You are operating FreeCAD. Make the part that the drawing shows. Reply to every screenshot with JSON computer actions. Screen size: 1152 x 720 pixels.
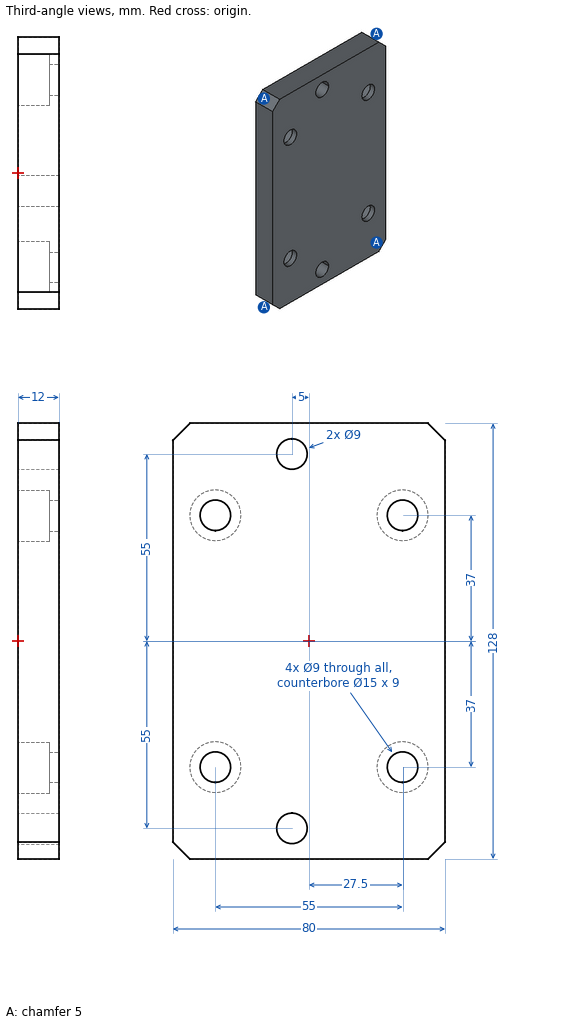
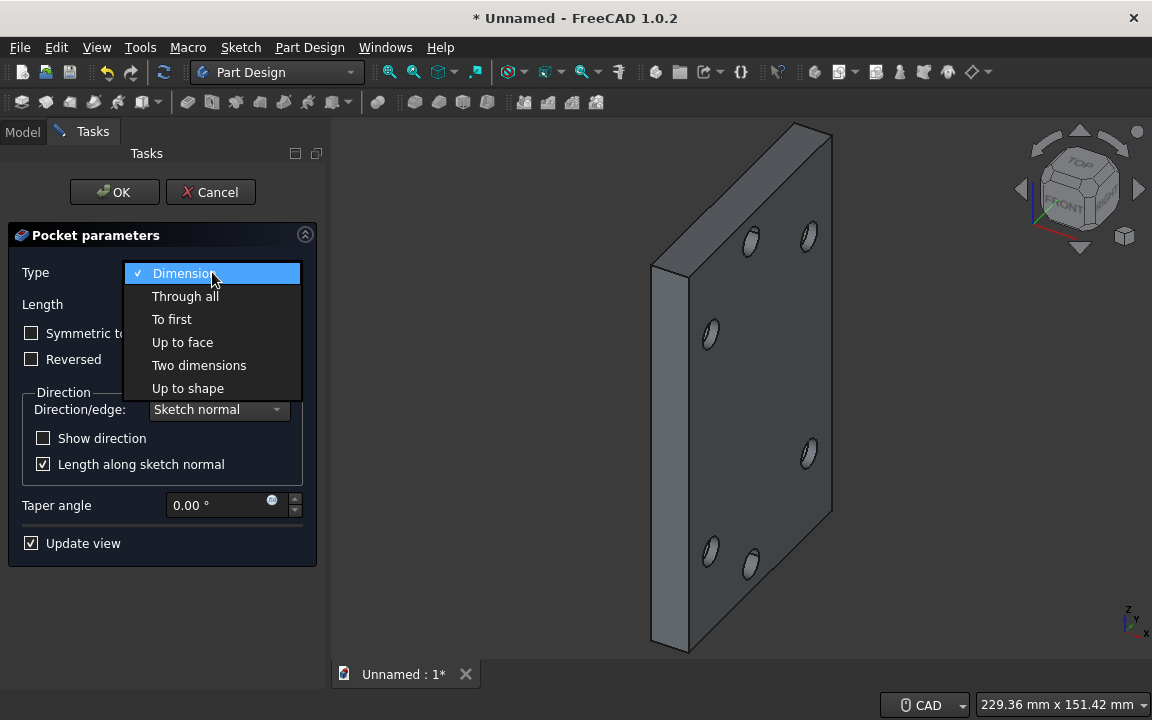
{"action": "left_click", "coordinate": [212, 296]}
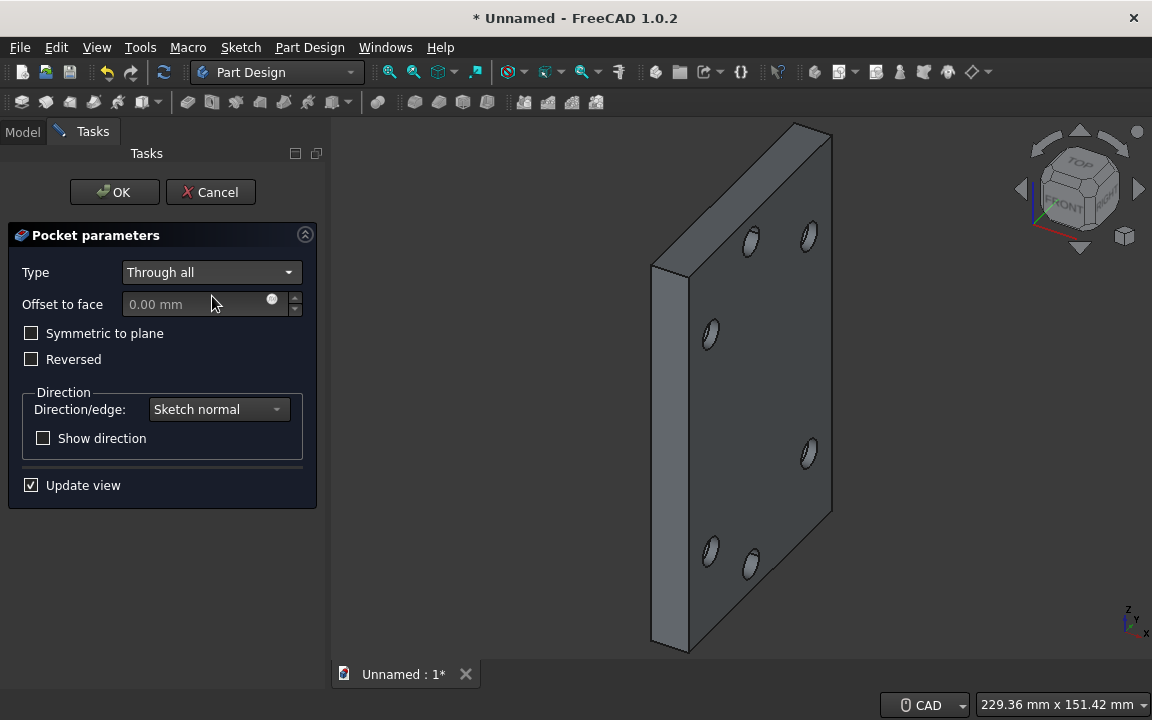
{"action": "left_click", "coordinate": [115, 192]}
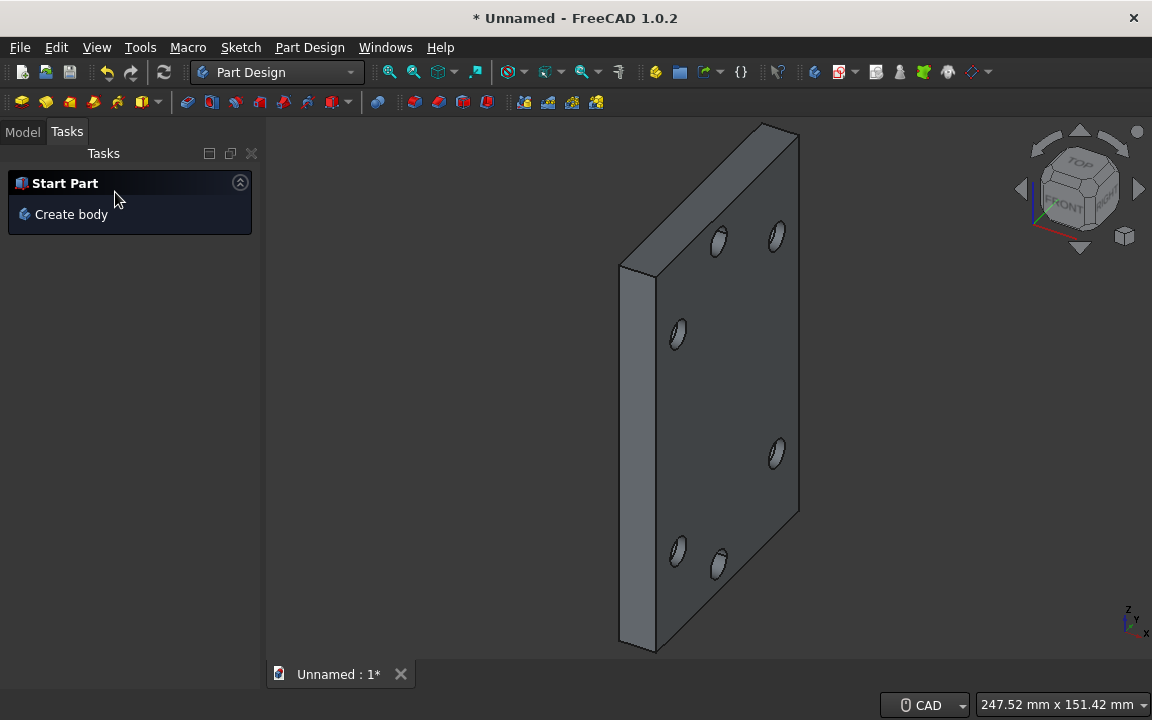
{"action": "left_click", "coordinate": [637, 270]}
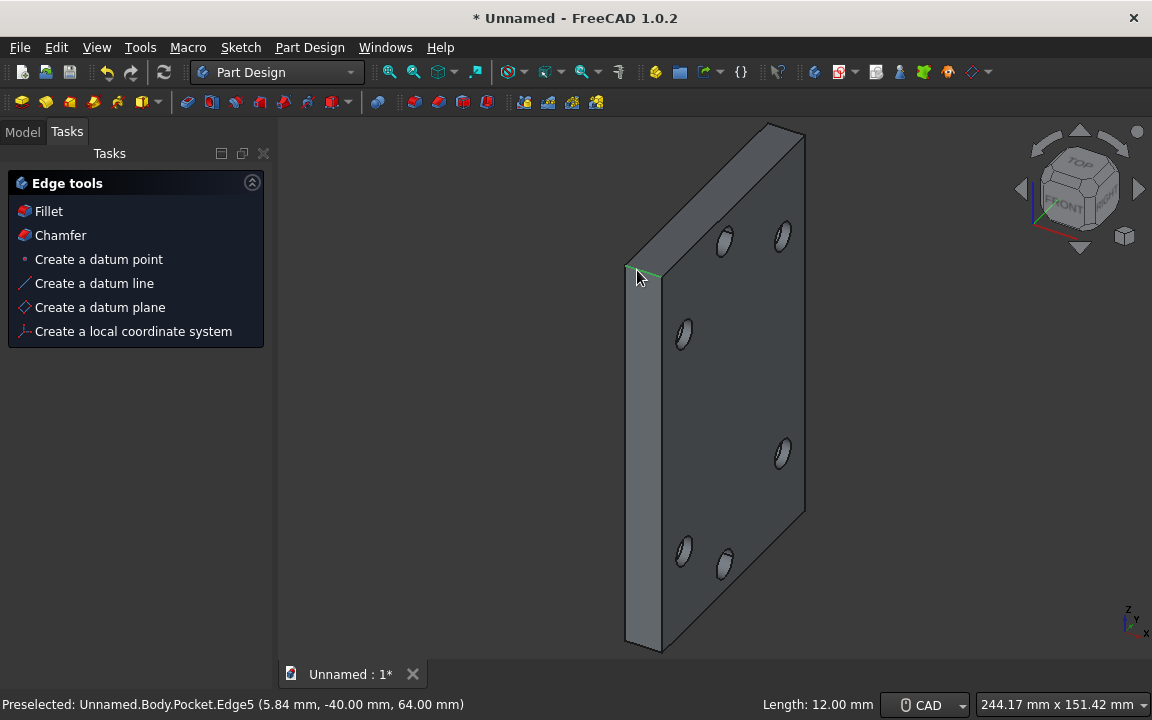
{"action": "key", "text": "0"}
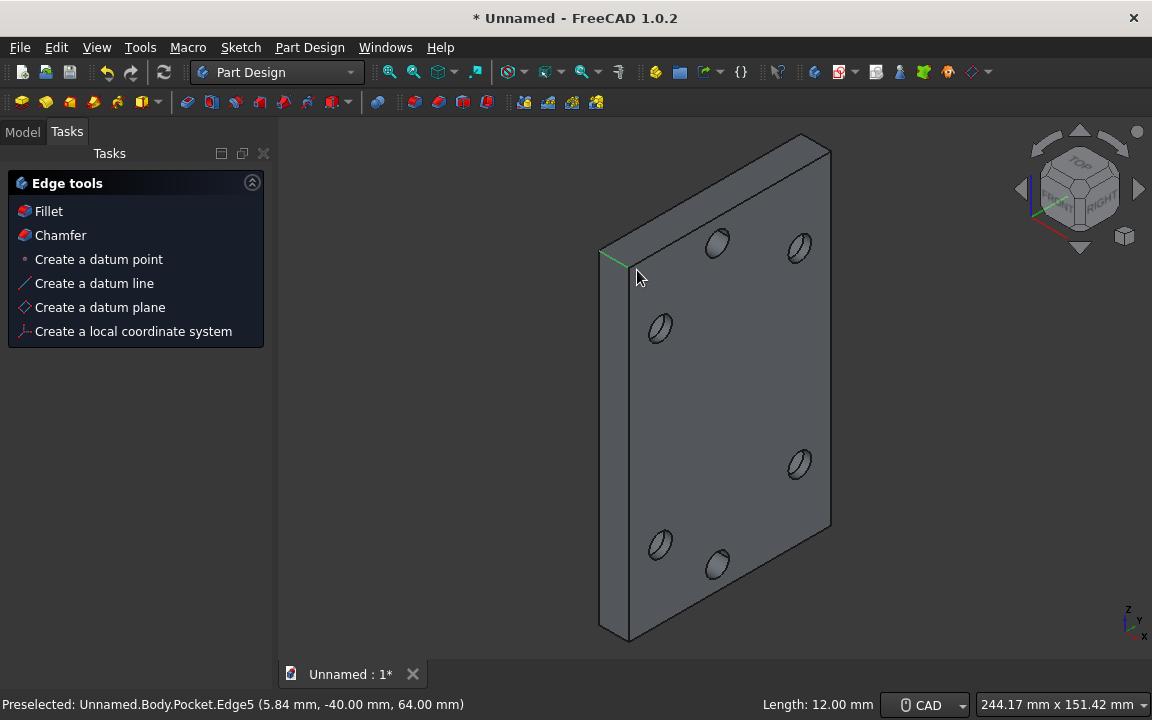
{"action": "key", "text": "2"}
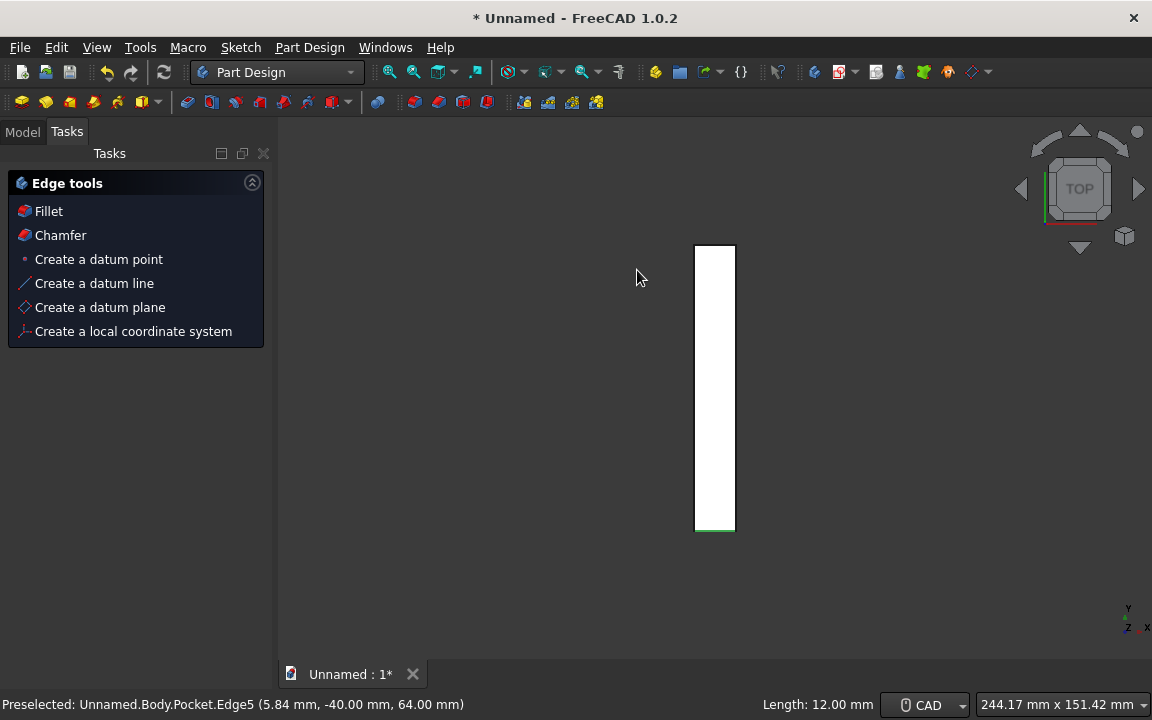
{"action": "left_click", "coordinate": [715, 244], "text": "ctrl"}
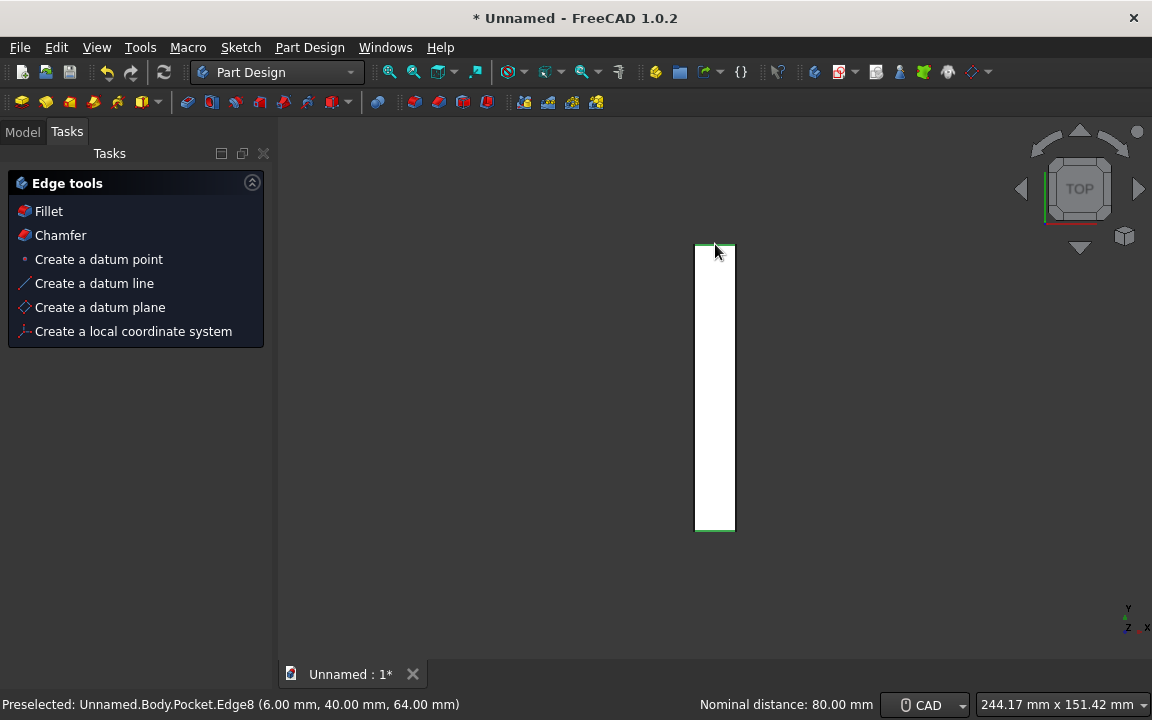
{"action": "key", "text": "1"}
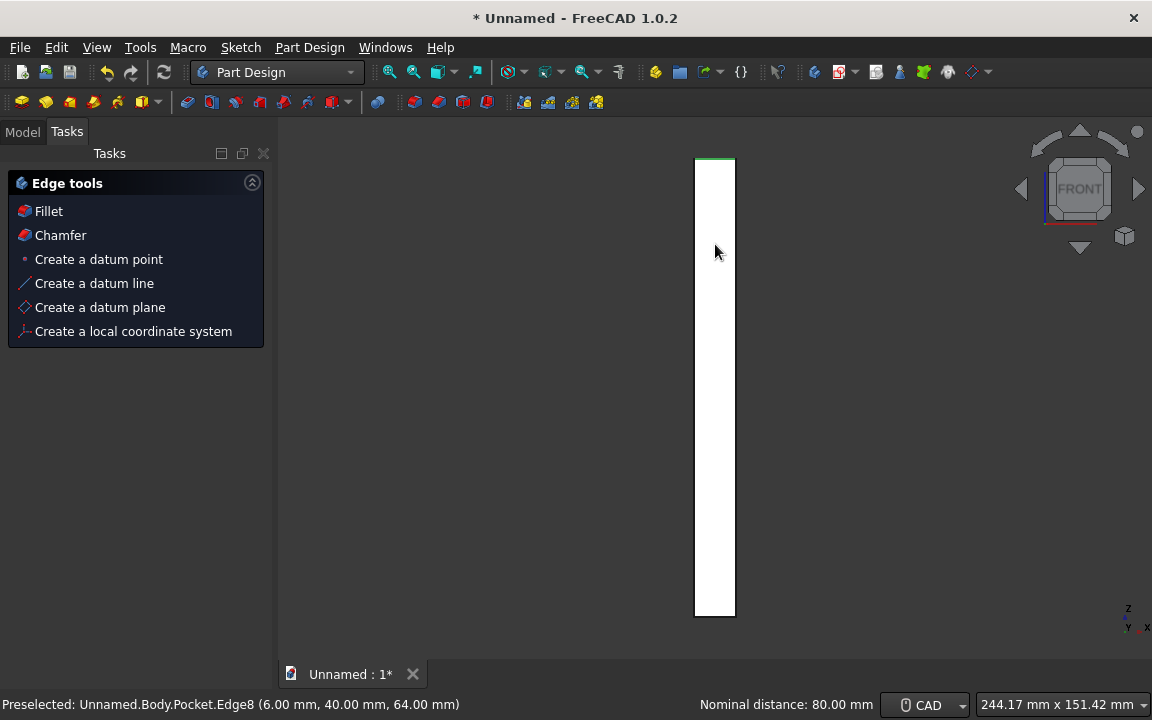
{"action": "left_click", "coordinate": [715, 616], "text": "ctrl"}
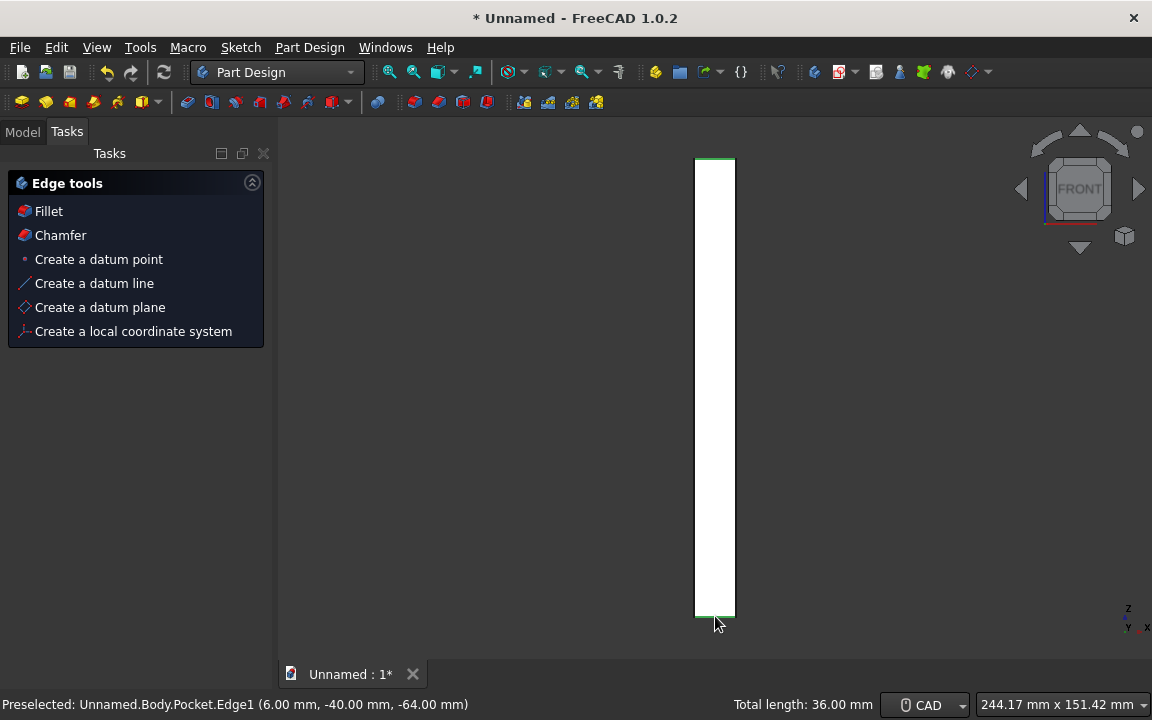
{"action": "key", "text": "3"}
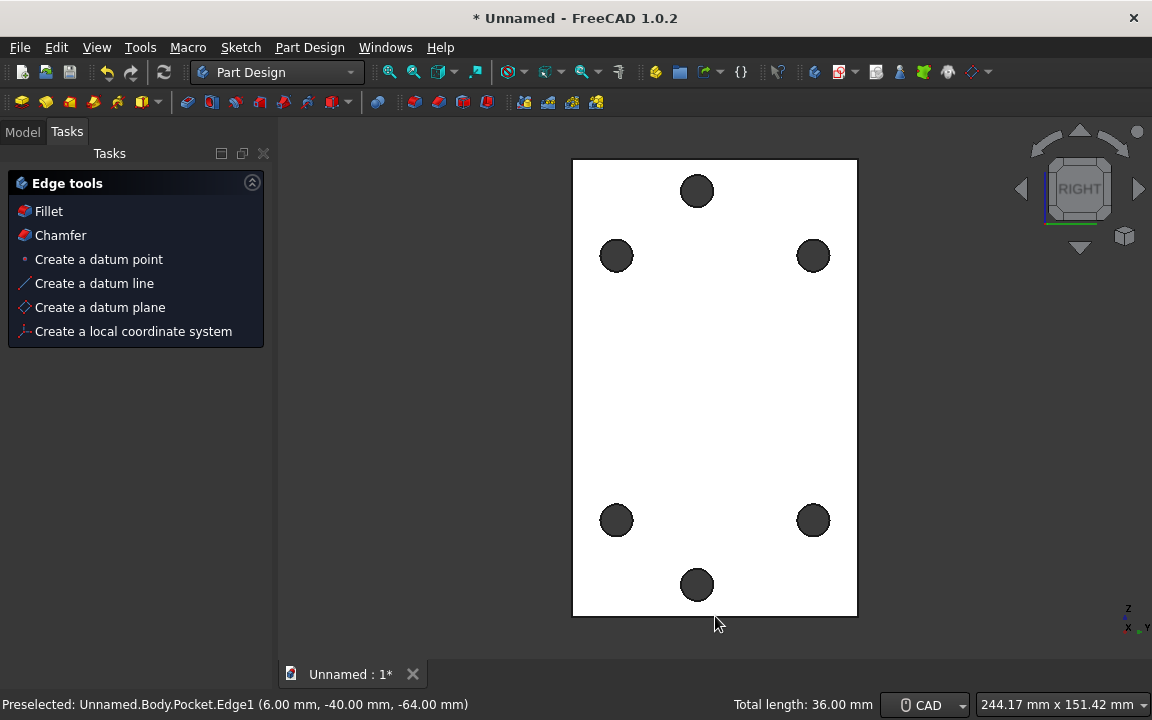
{"action": "key", "text": "5"}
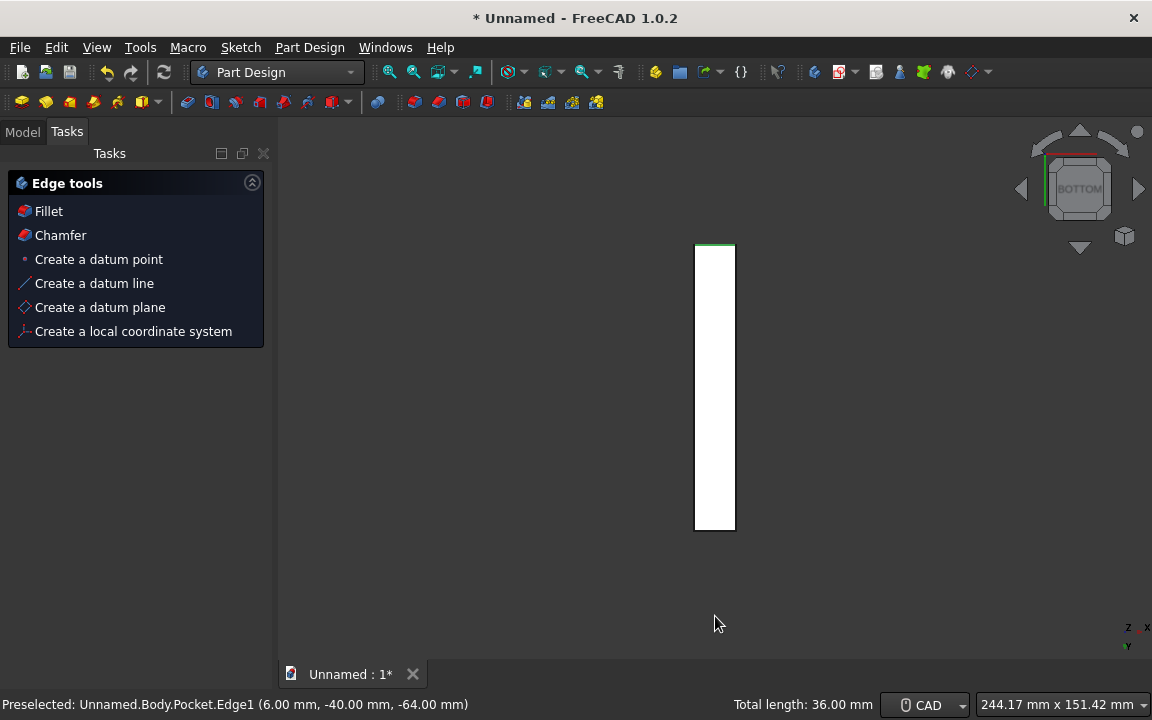
{"action": "left_click", "coordinate": [715, 530], "text": "ctrl"}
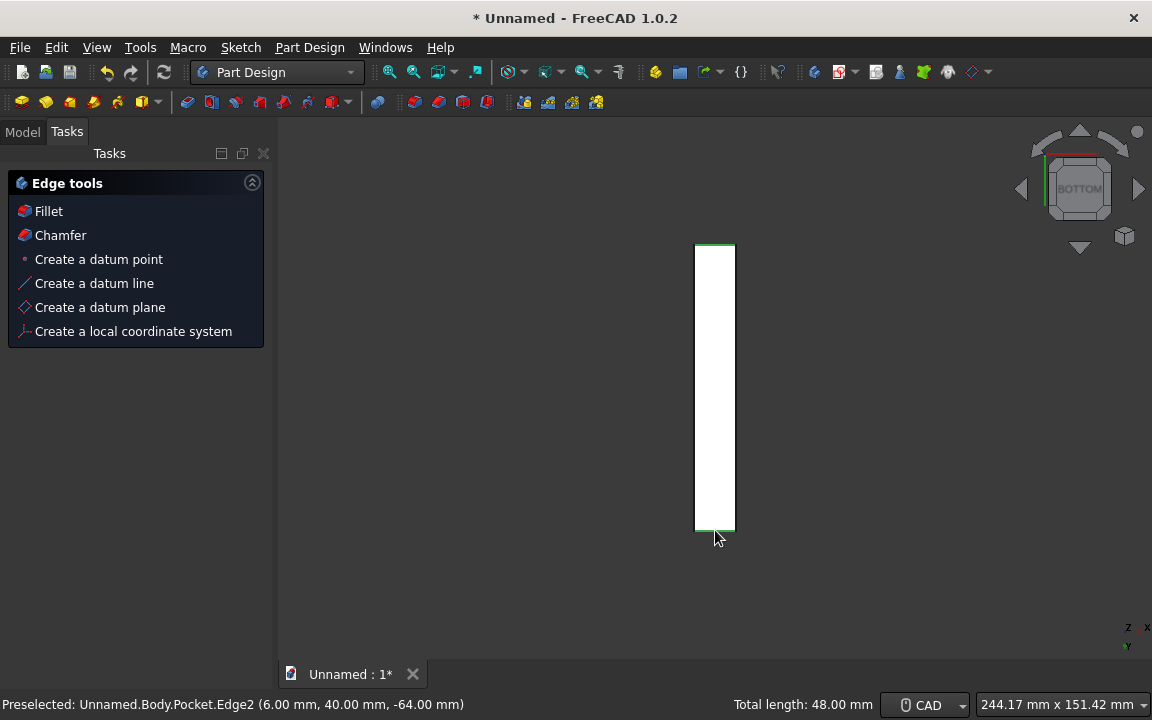
{"action": "left_click", "coordinate": [440, 102]}